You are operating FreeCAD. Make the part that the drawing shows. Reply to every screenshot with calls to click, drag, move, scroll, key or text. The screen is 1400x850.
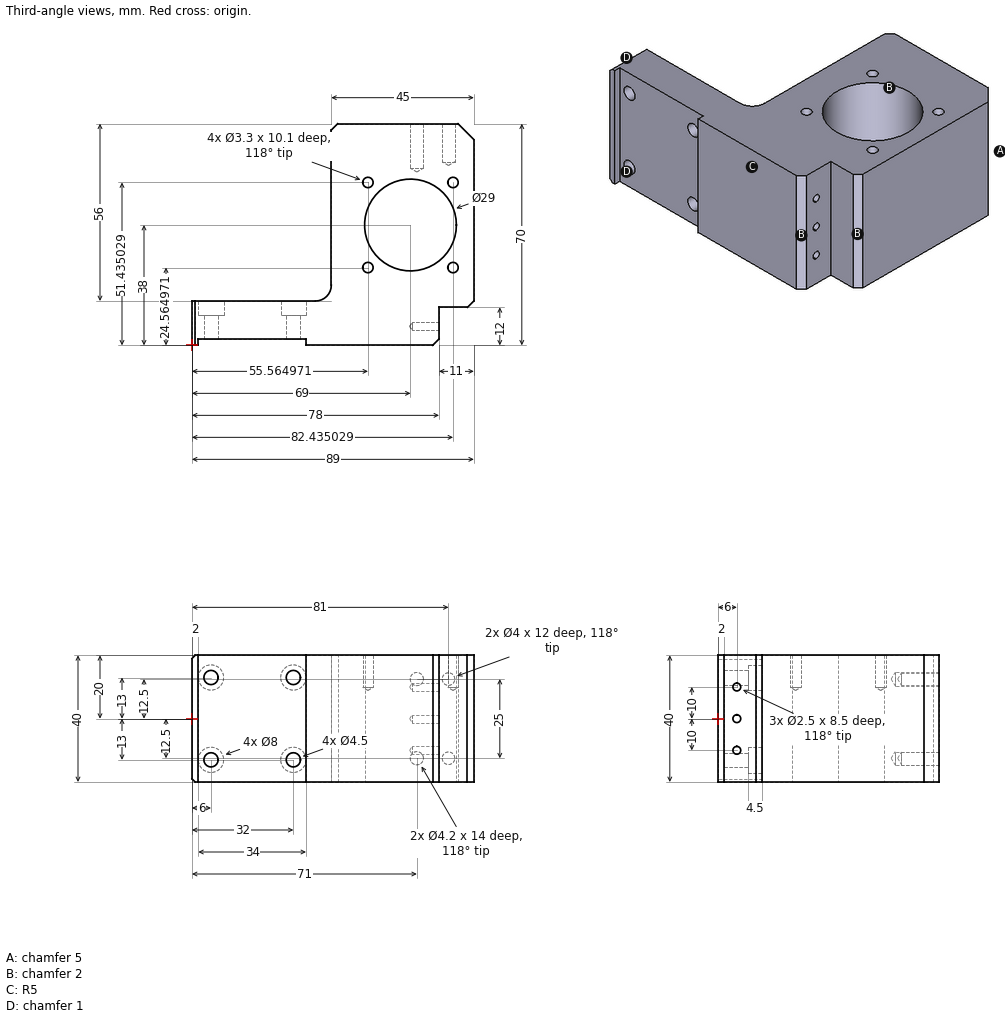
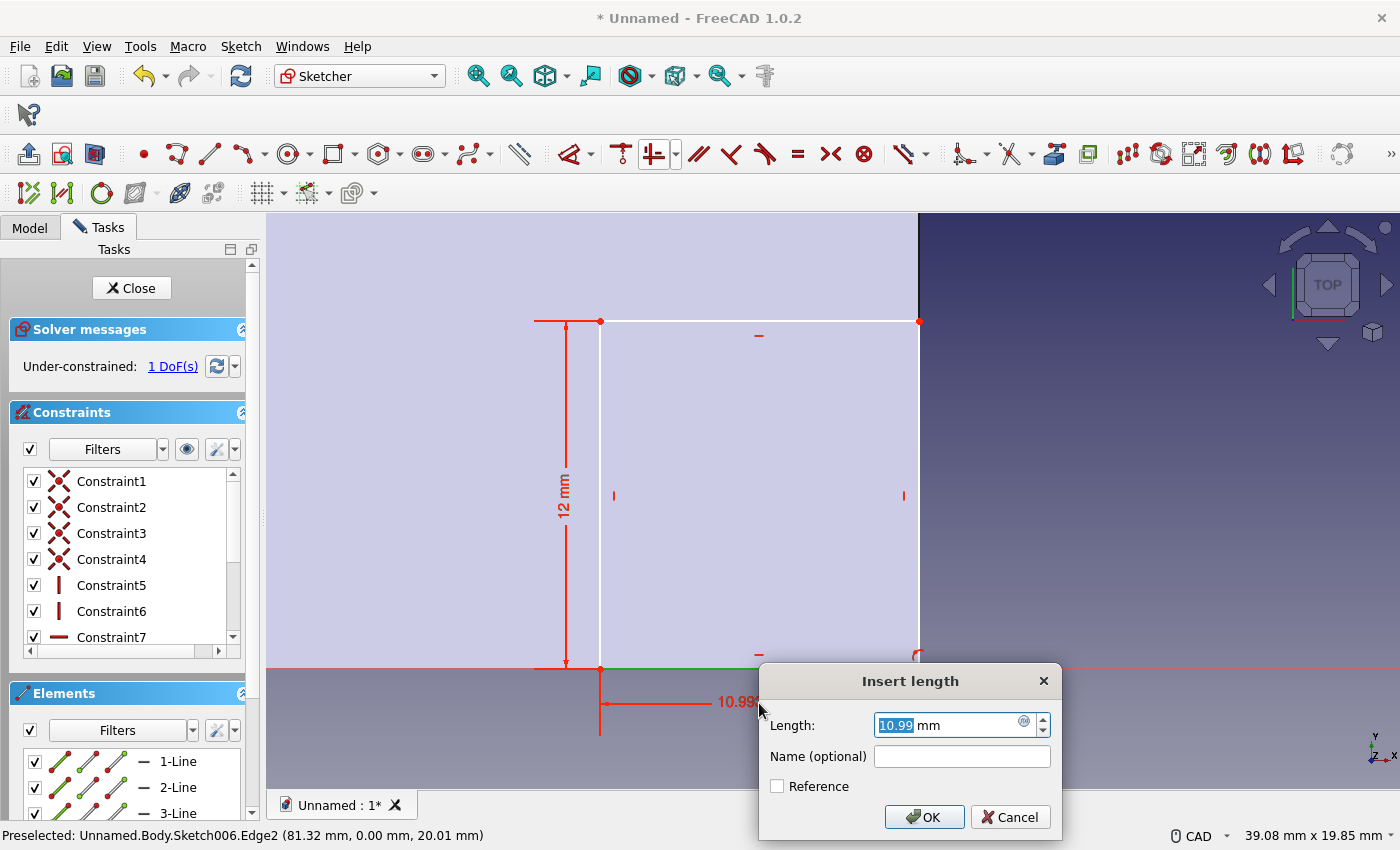
text(11)
key(Return)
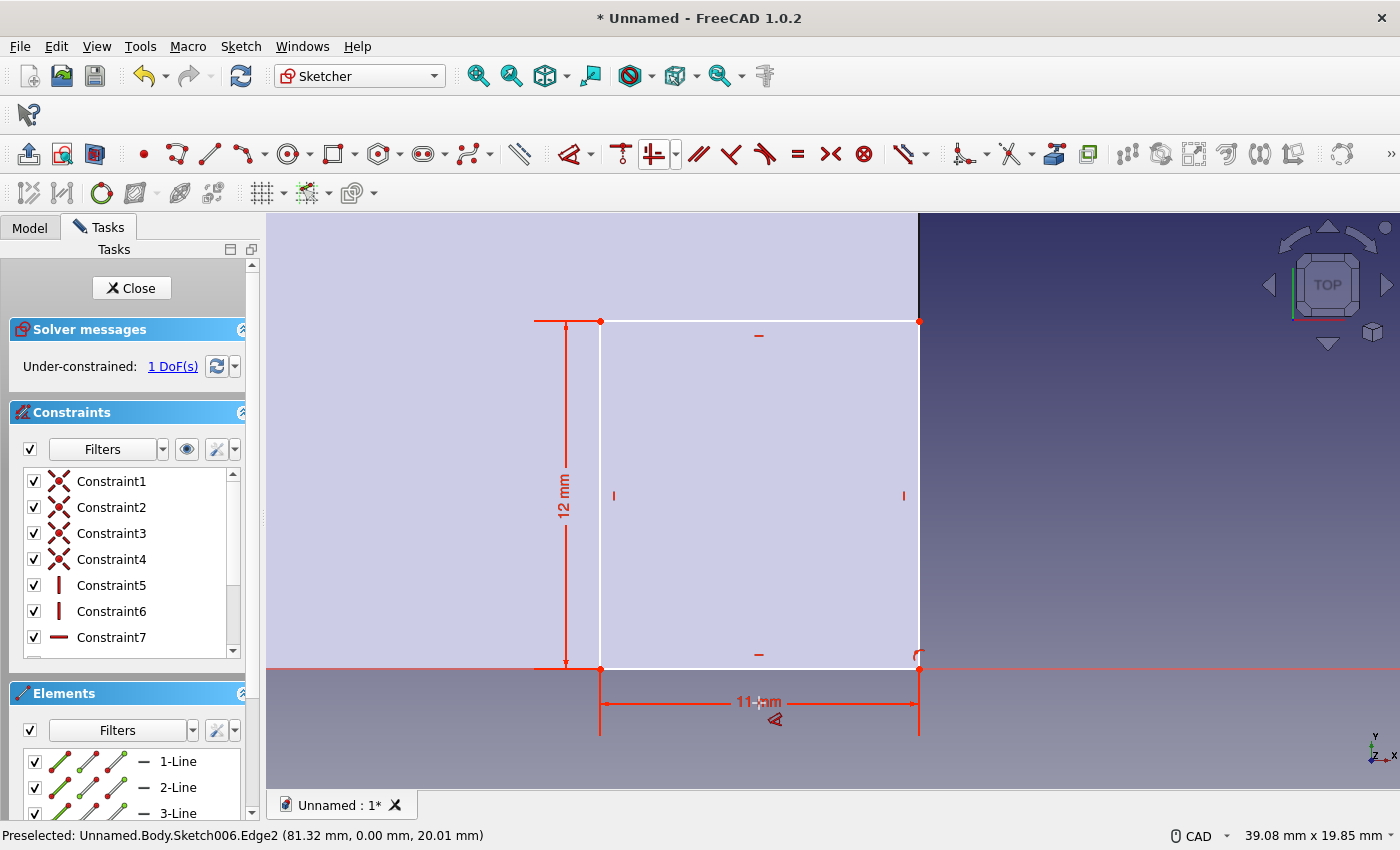
click(600, 321)
click(447, 703)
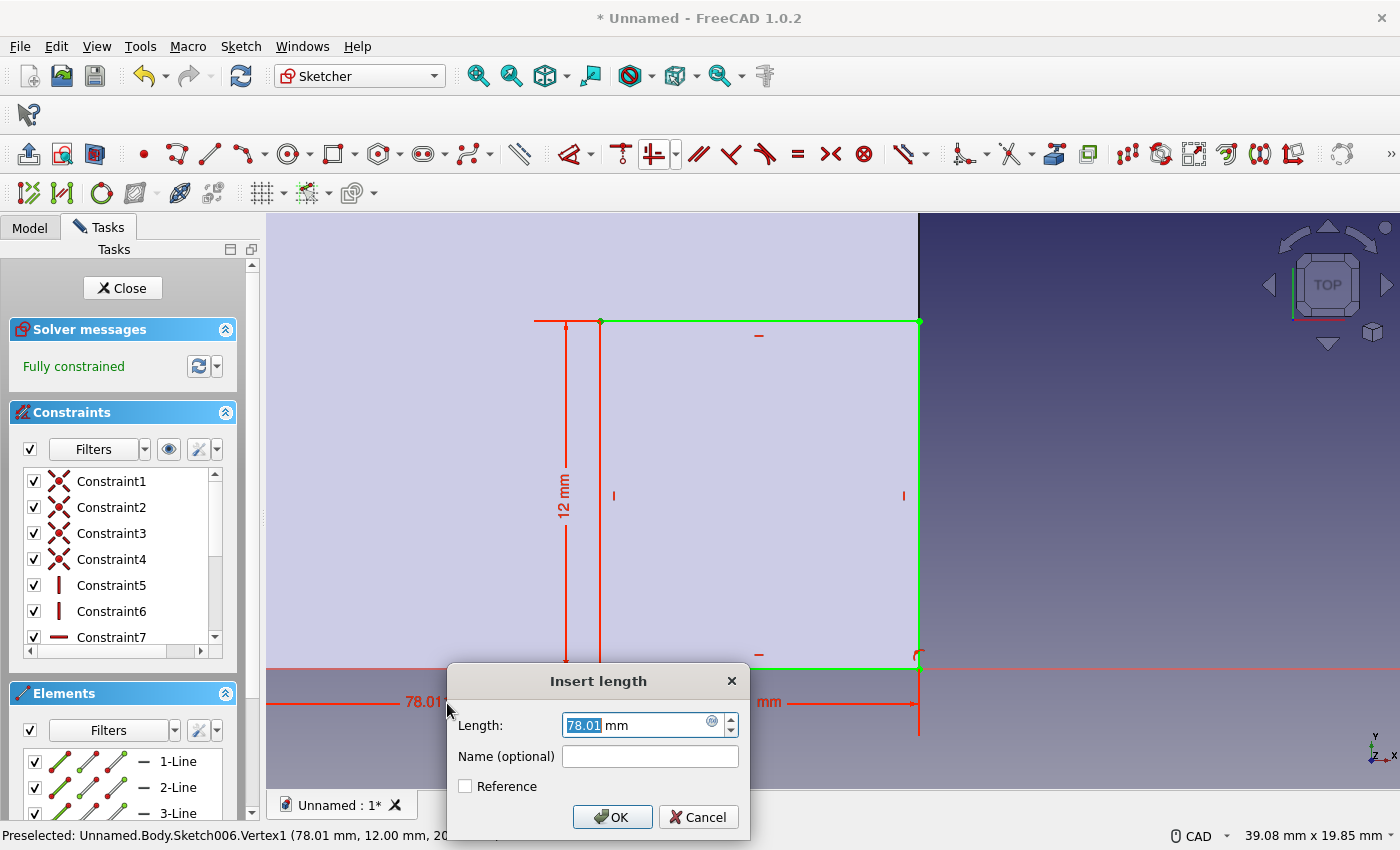
text(78)
key(Return)
key(Escape)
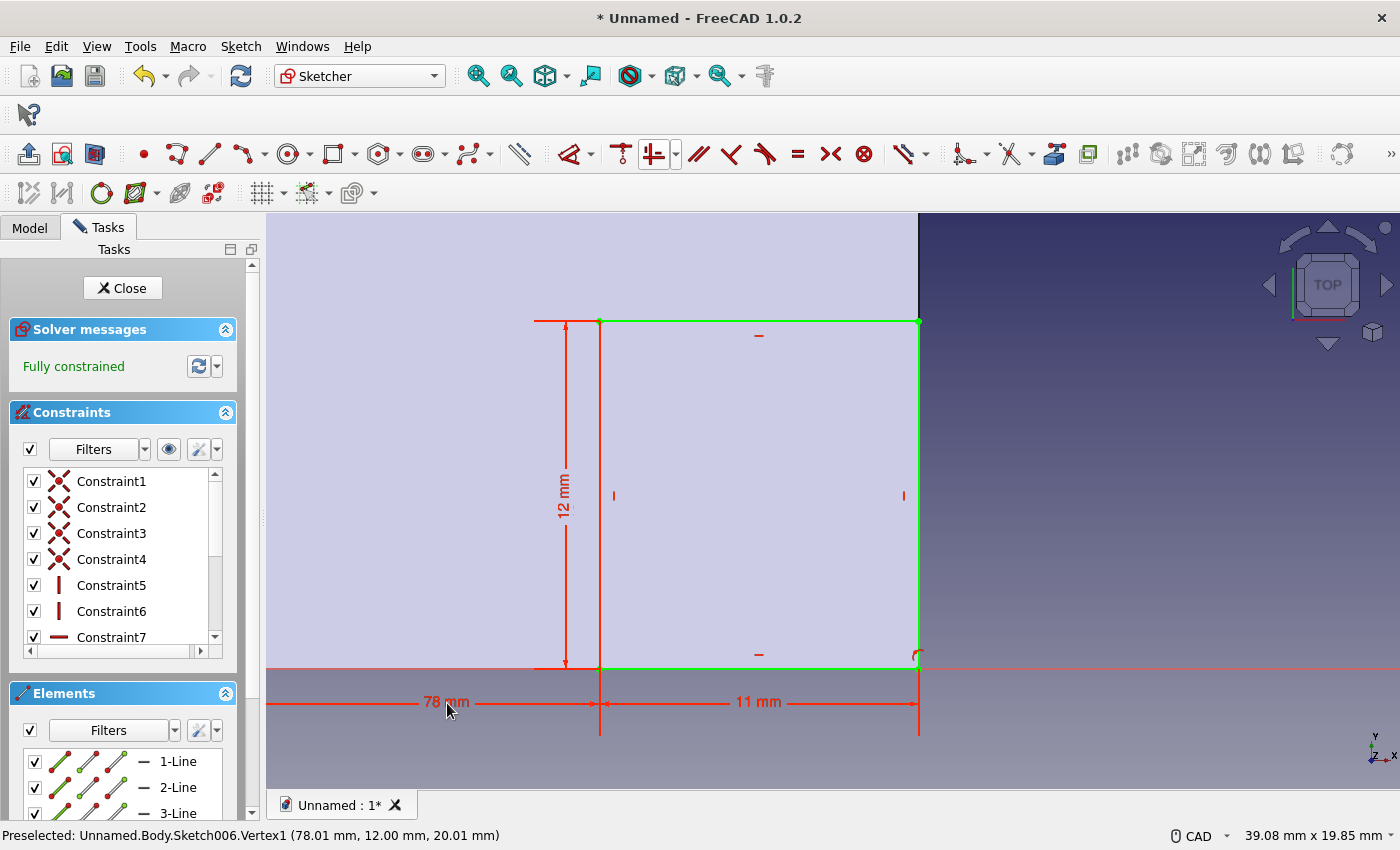
click(123, 288)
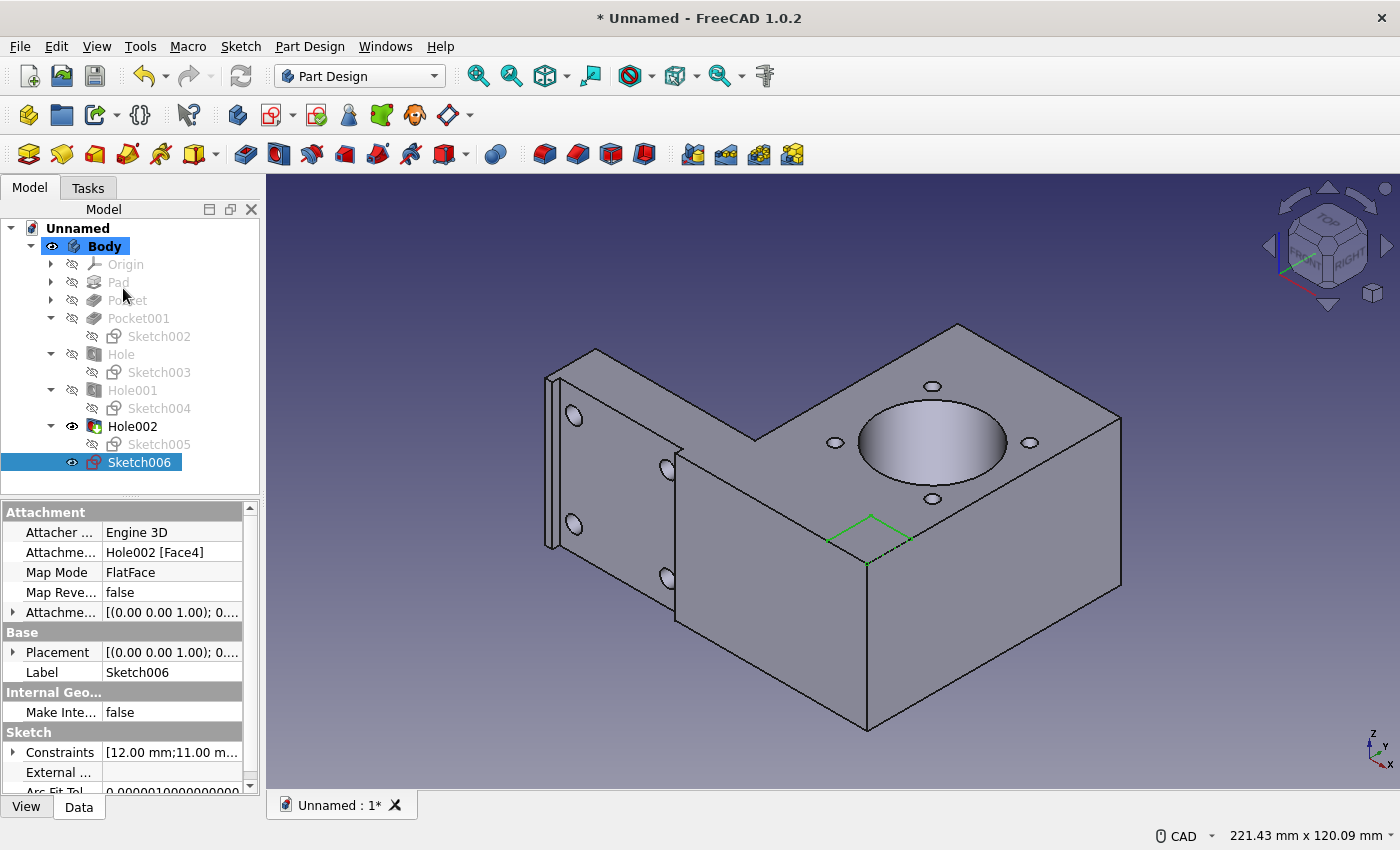
click(246, 154)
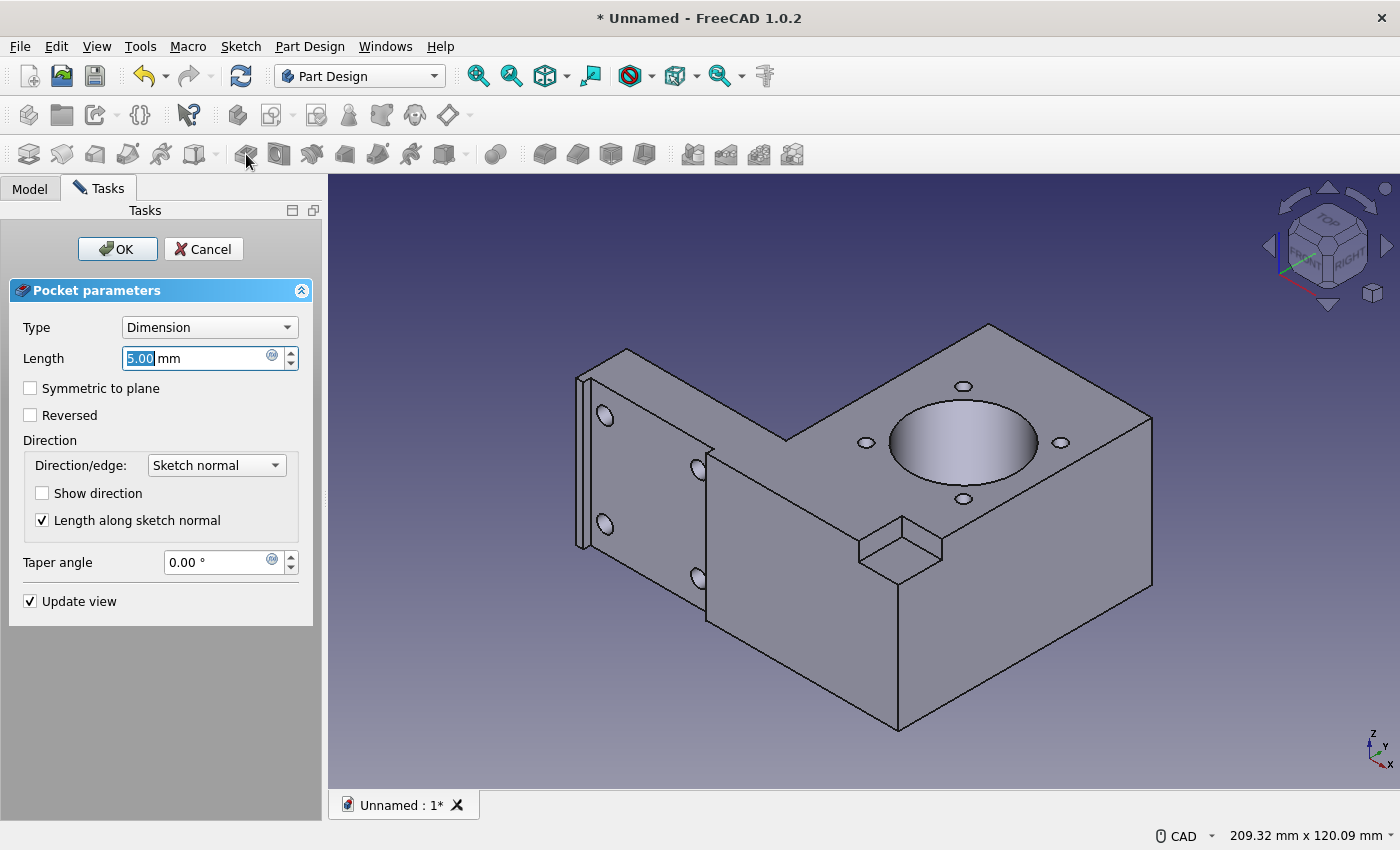
click(210, 328)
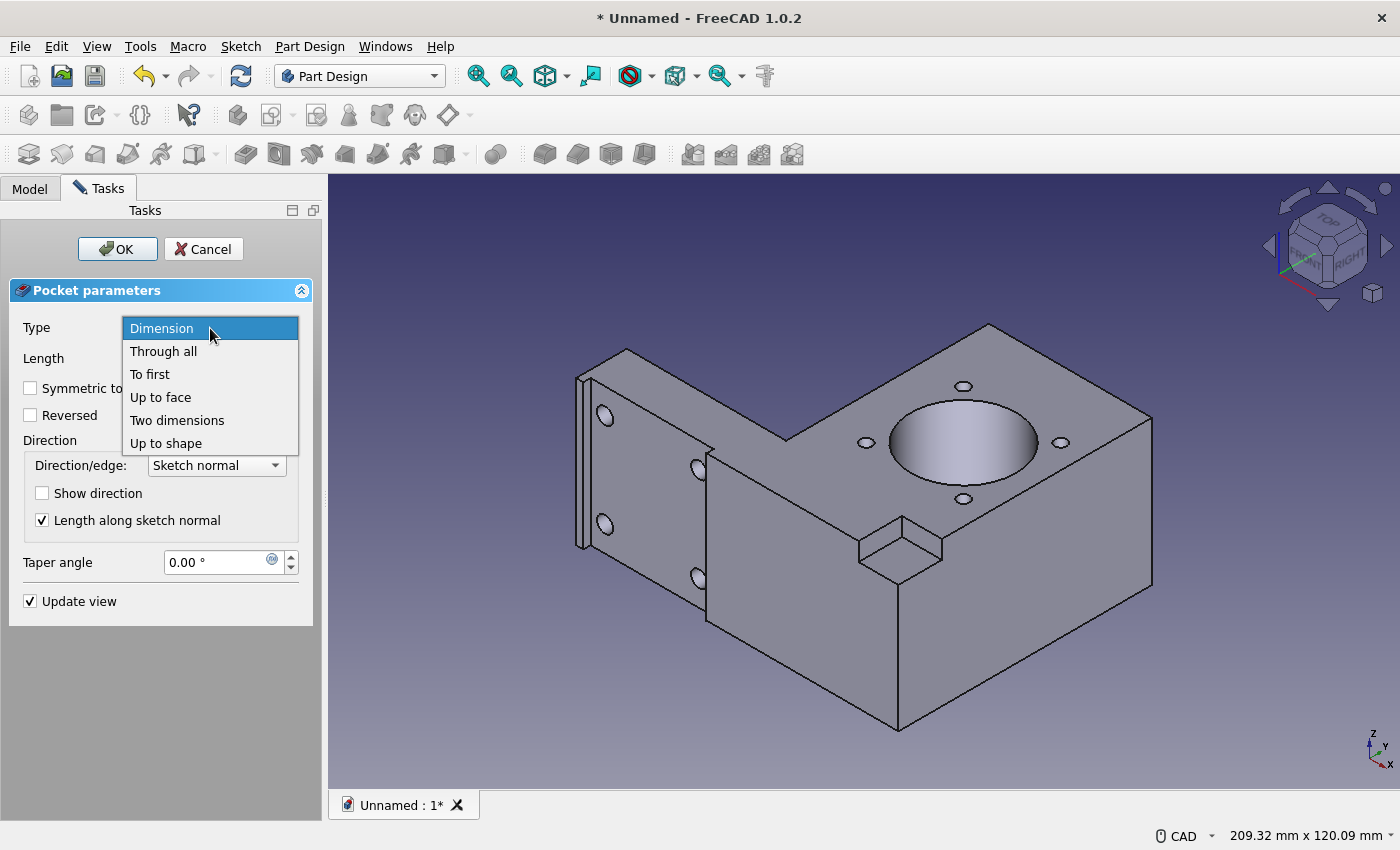
click(208, 352)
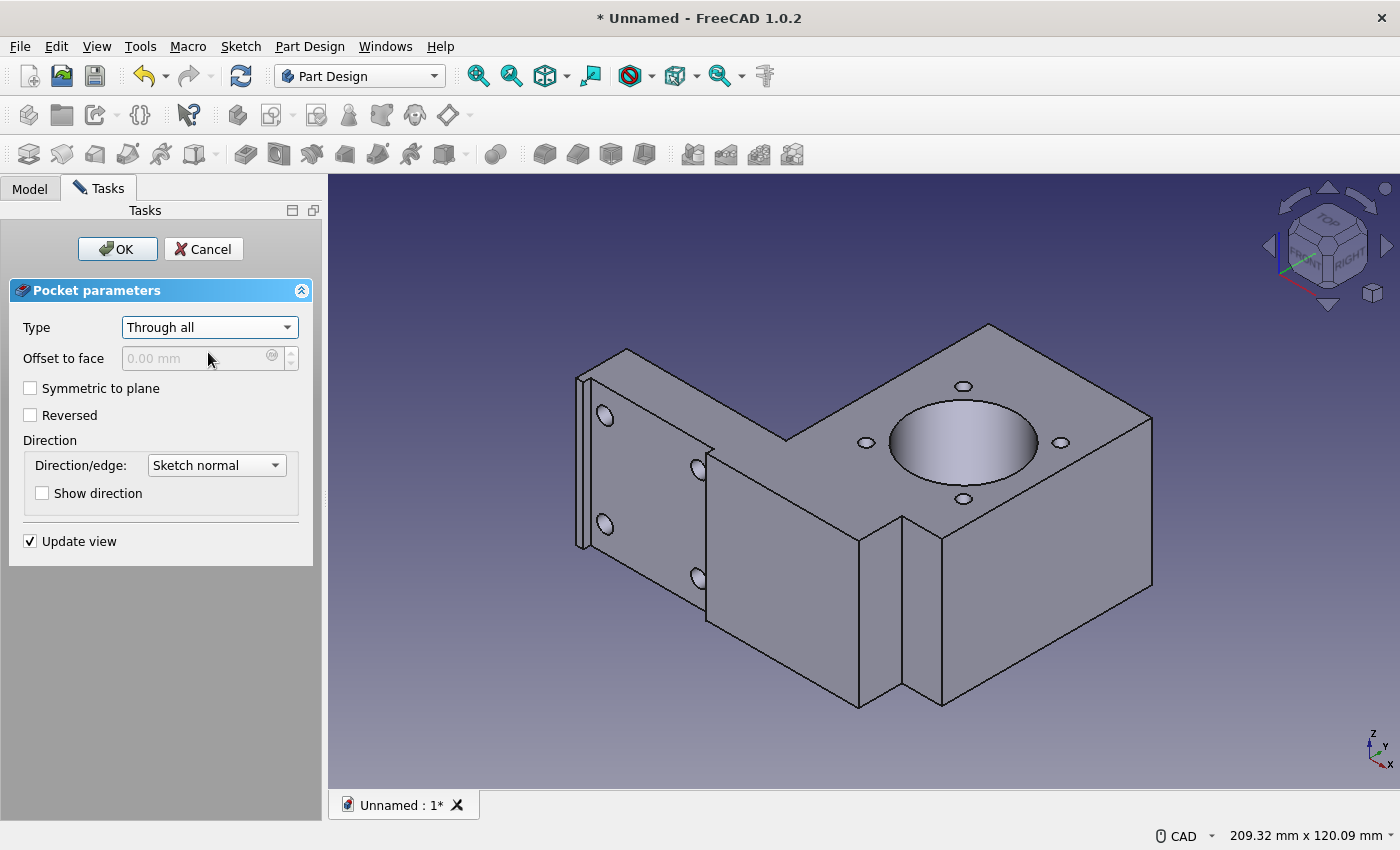
click(118, 249)